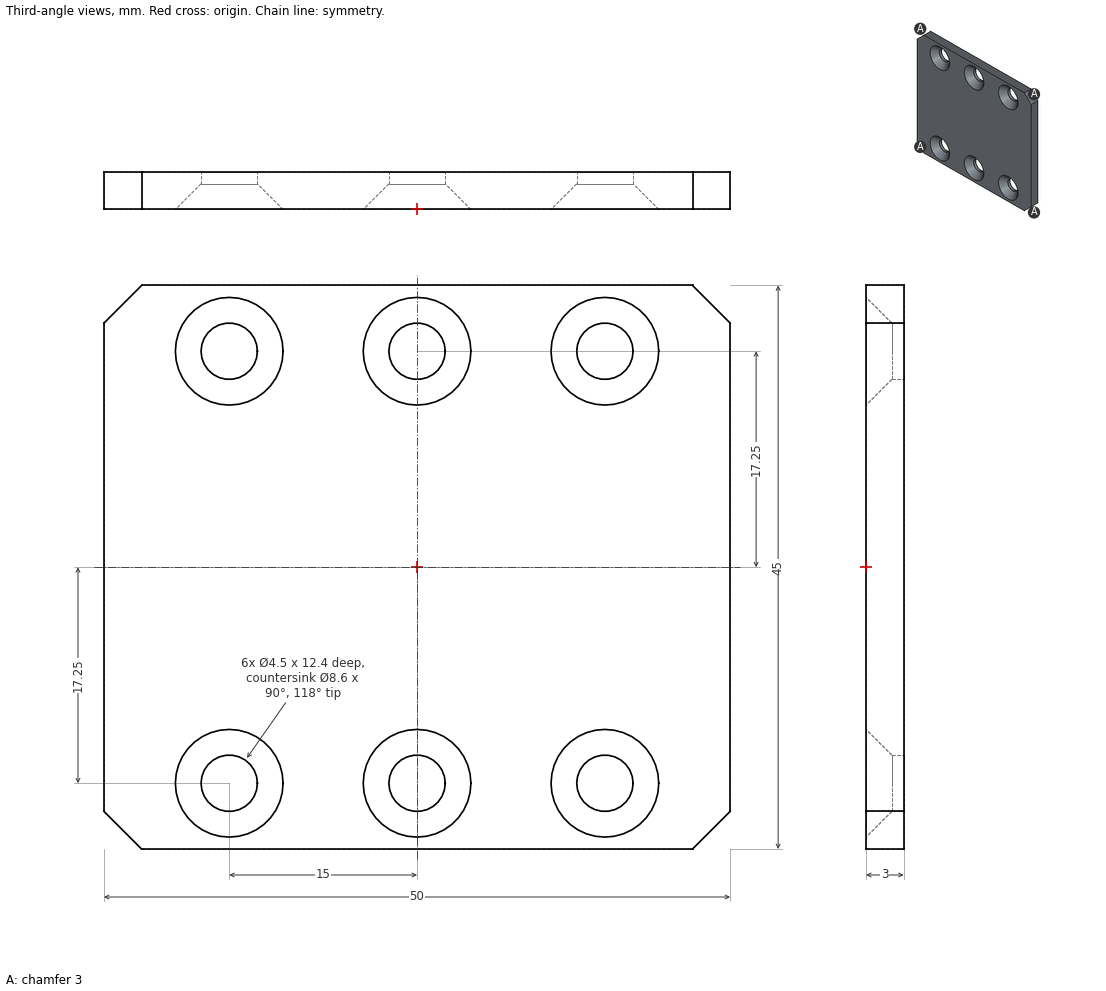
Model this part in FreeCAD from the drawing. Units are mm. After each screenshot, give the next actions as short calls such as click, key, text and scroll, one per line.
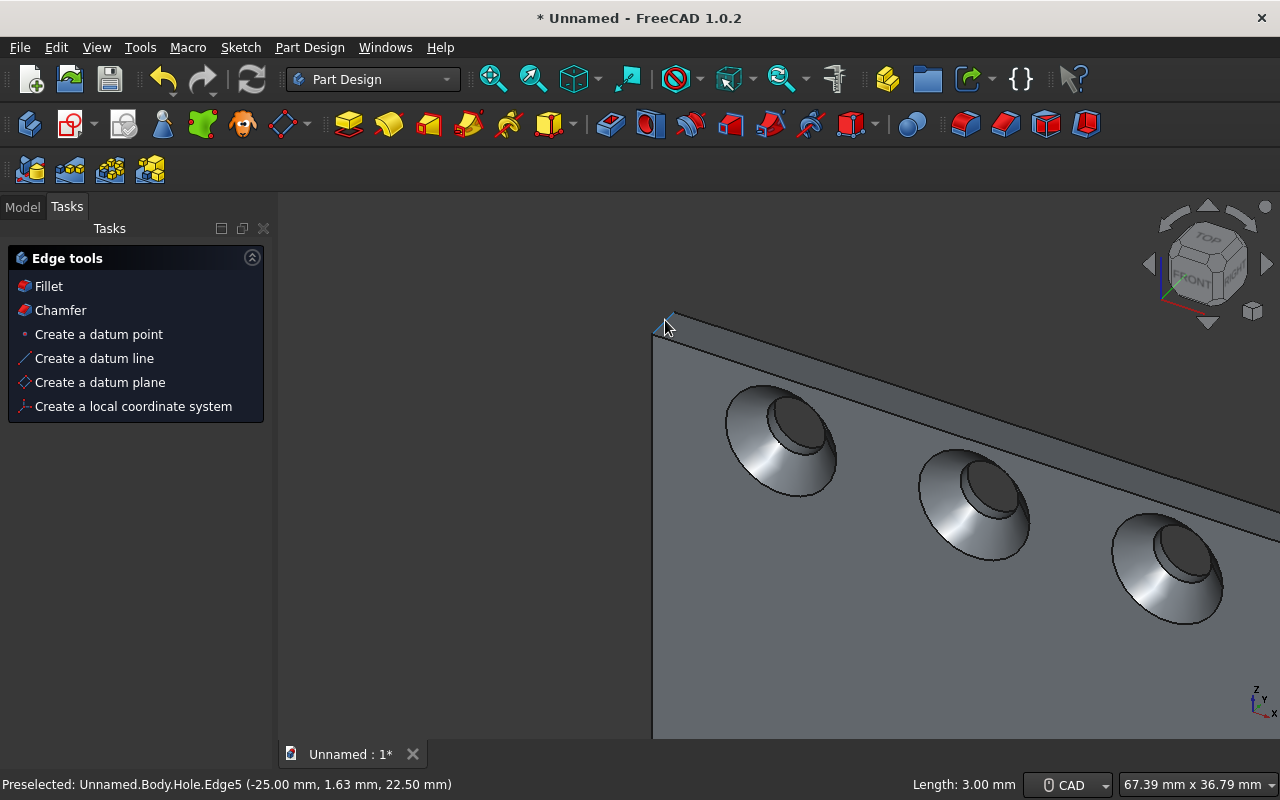
key(v)
key(f)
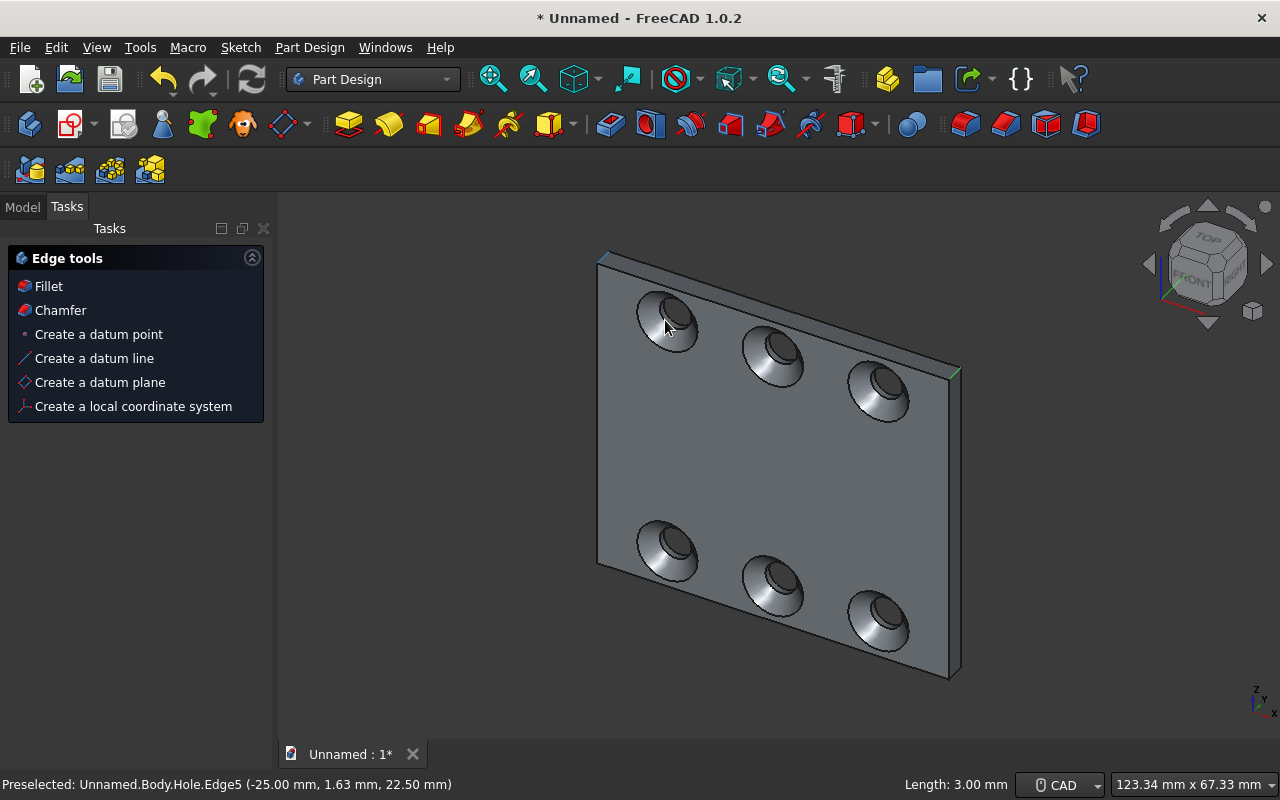
key(0)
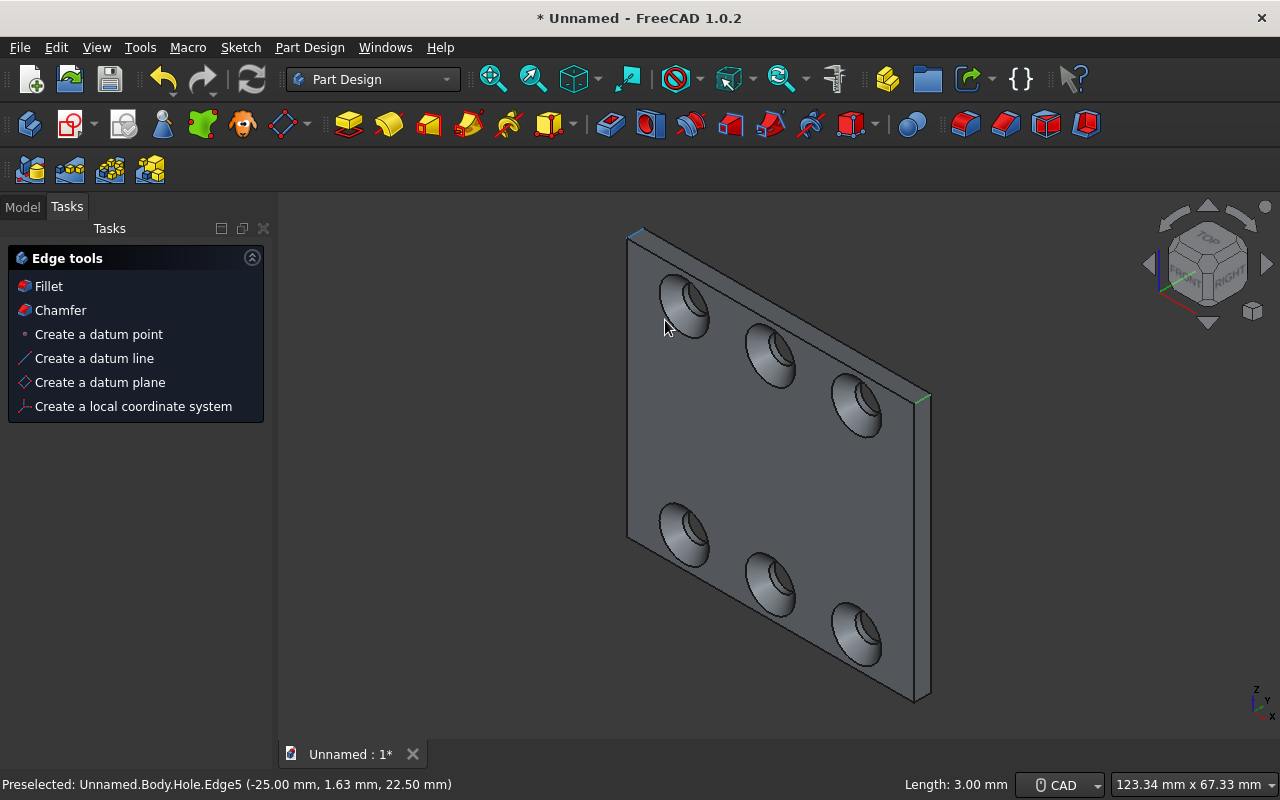
key(2)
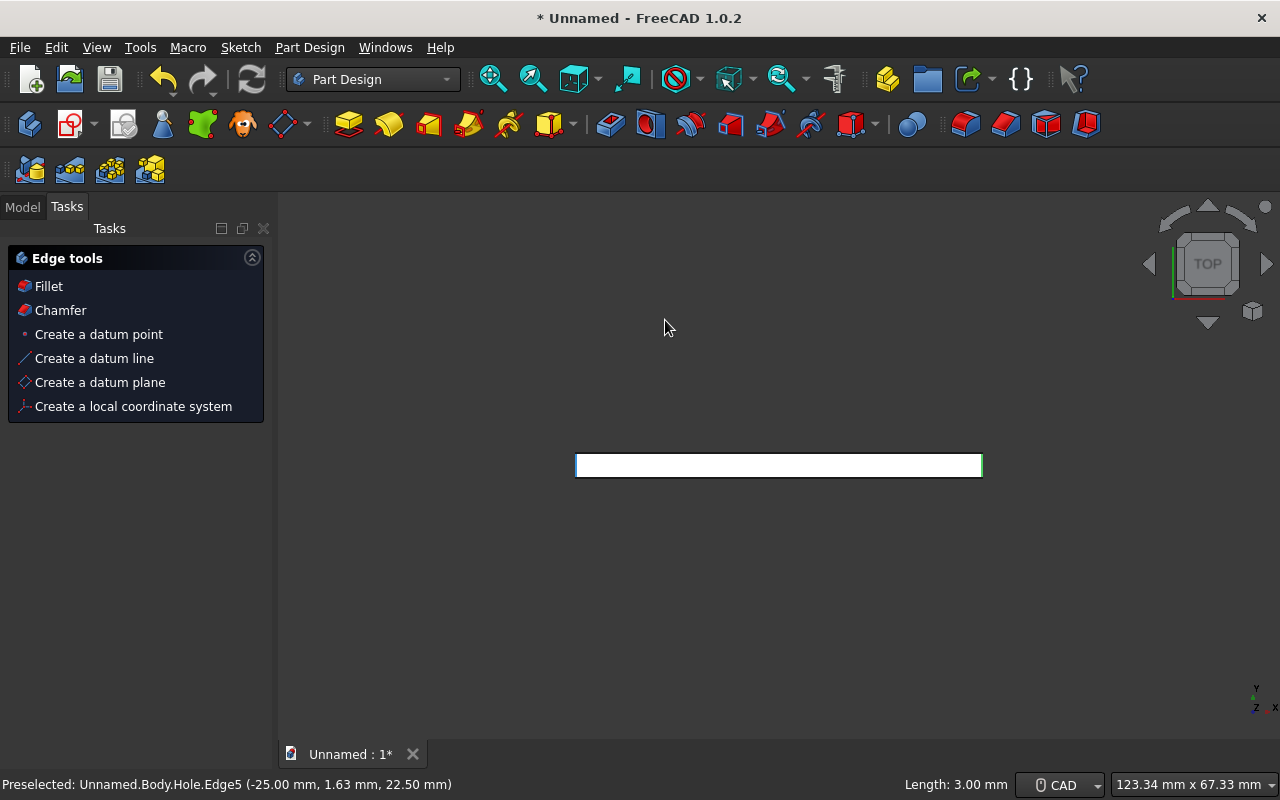
click(494, 80)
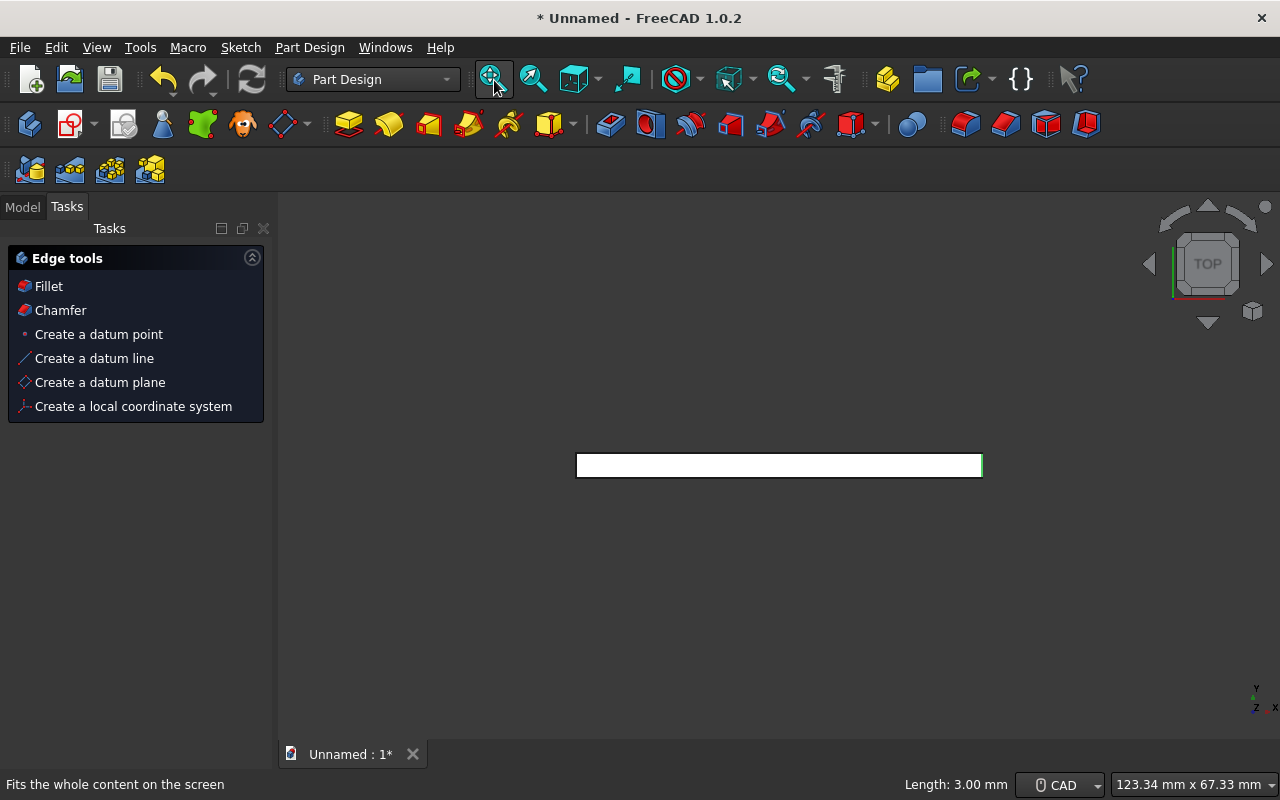
click(576, 464, ctrl)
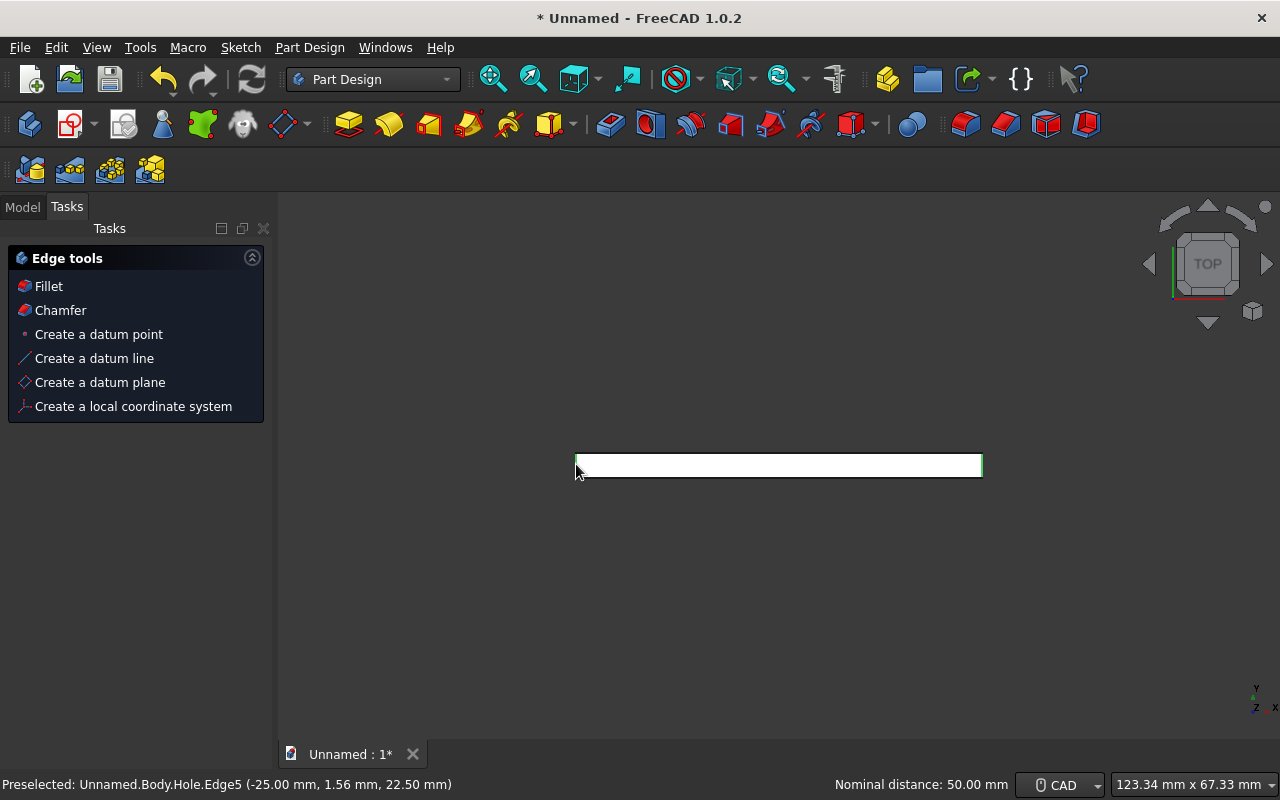
key(1)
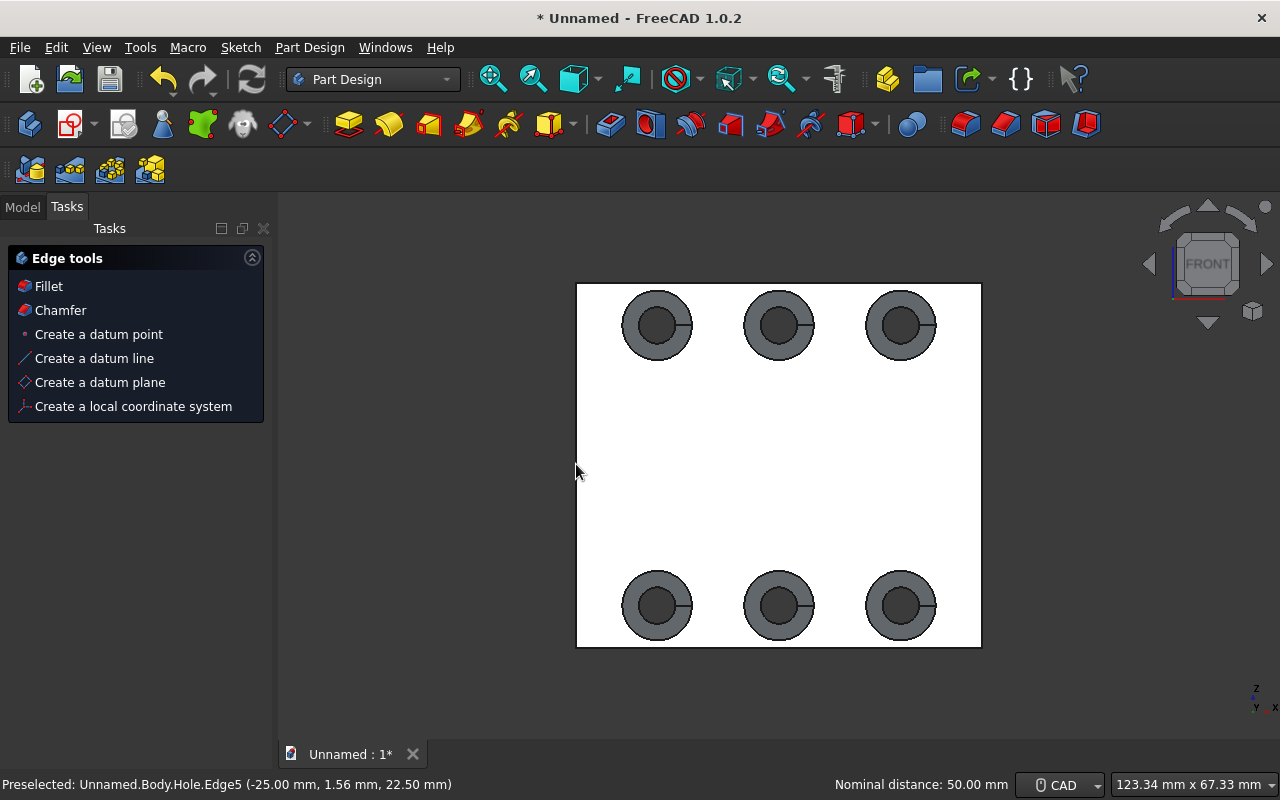
key(3)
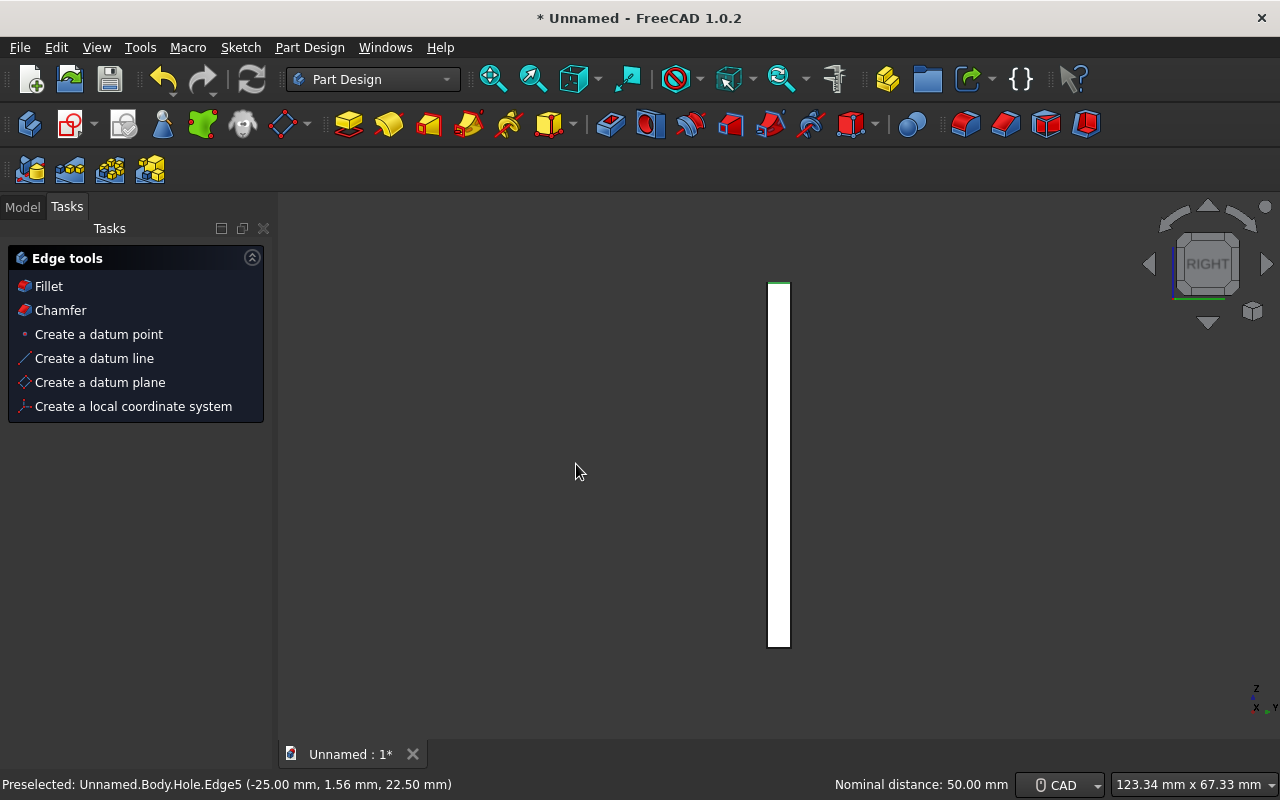
click(779, 647, ctrl)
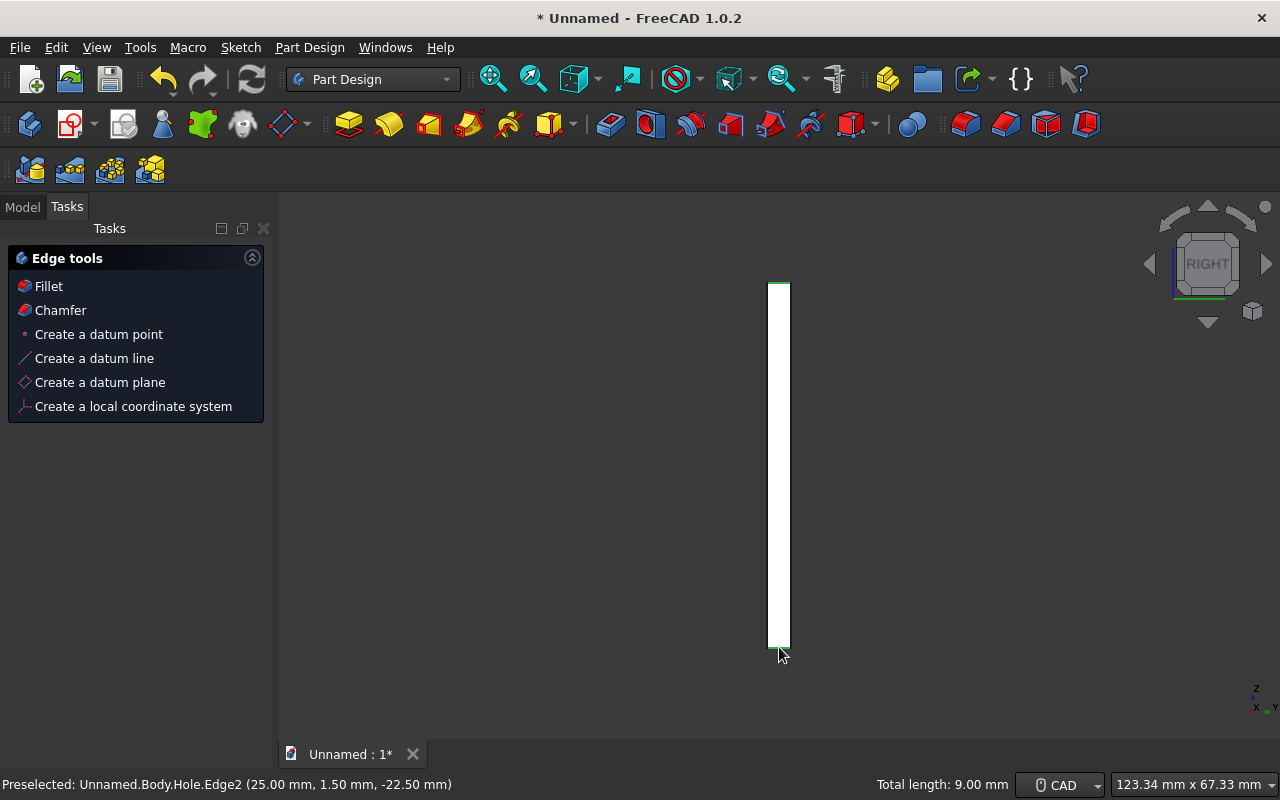
key(5)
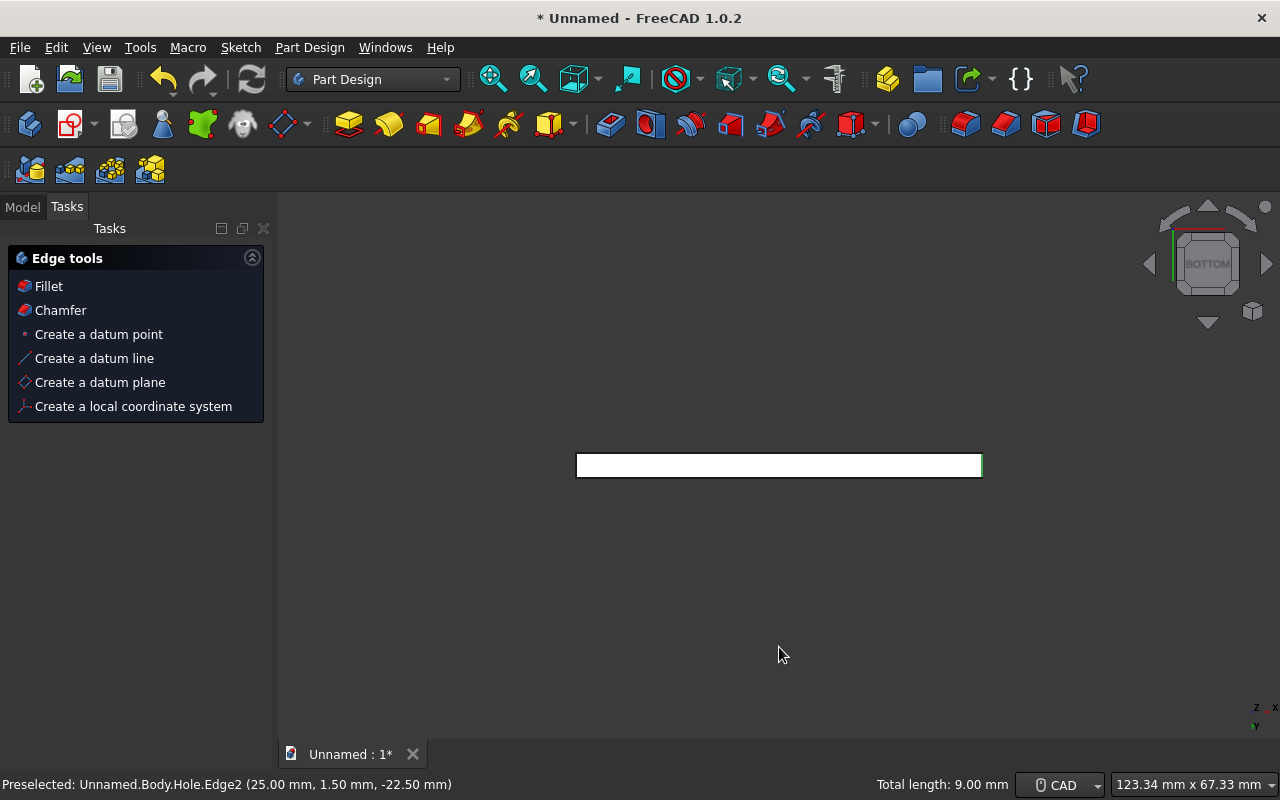
key(v)
key(f)